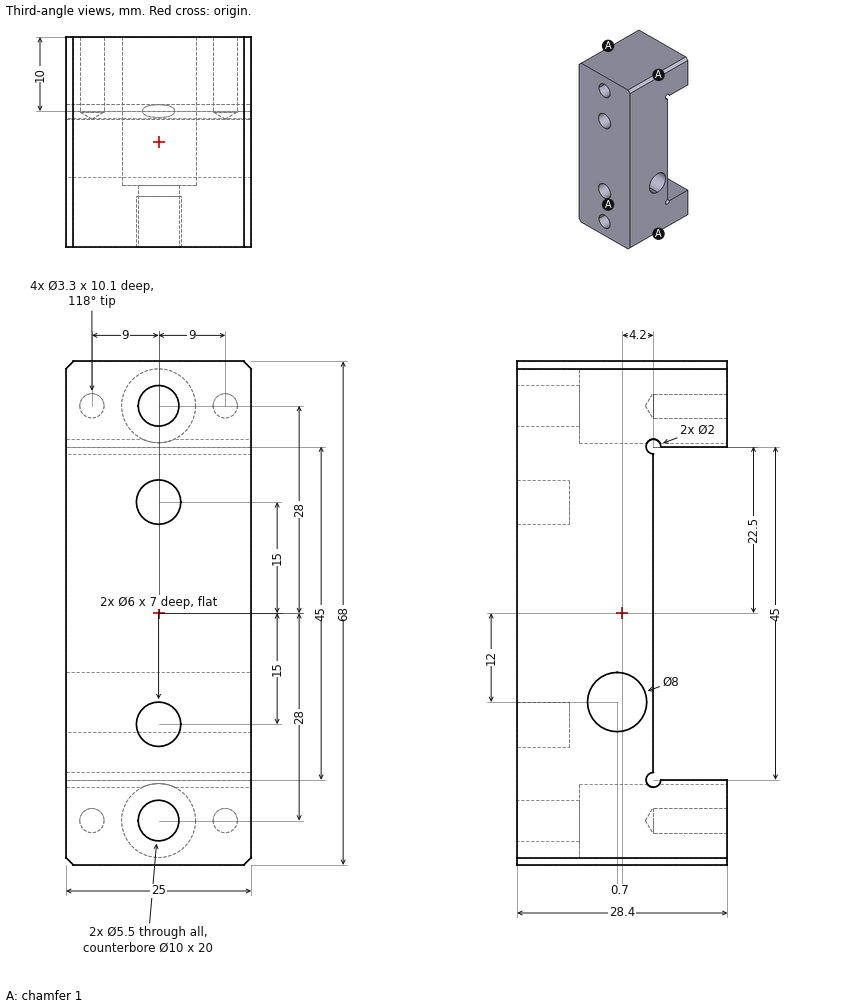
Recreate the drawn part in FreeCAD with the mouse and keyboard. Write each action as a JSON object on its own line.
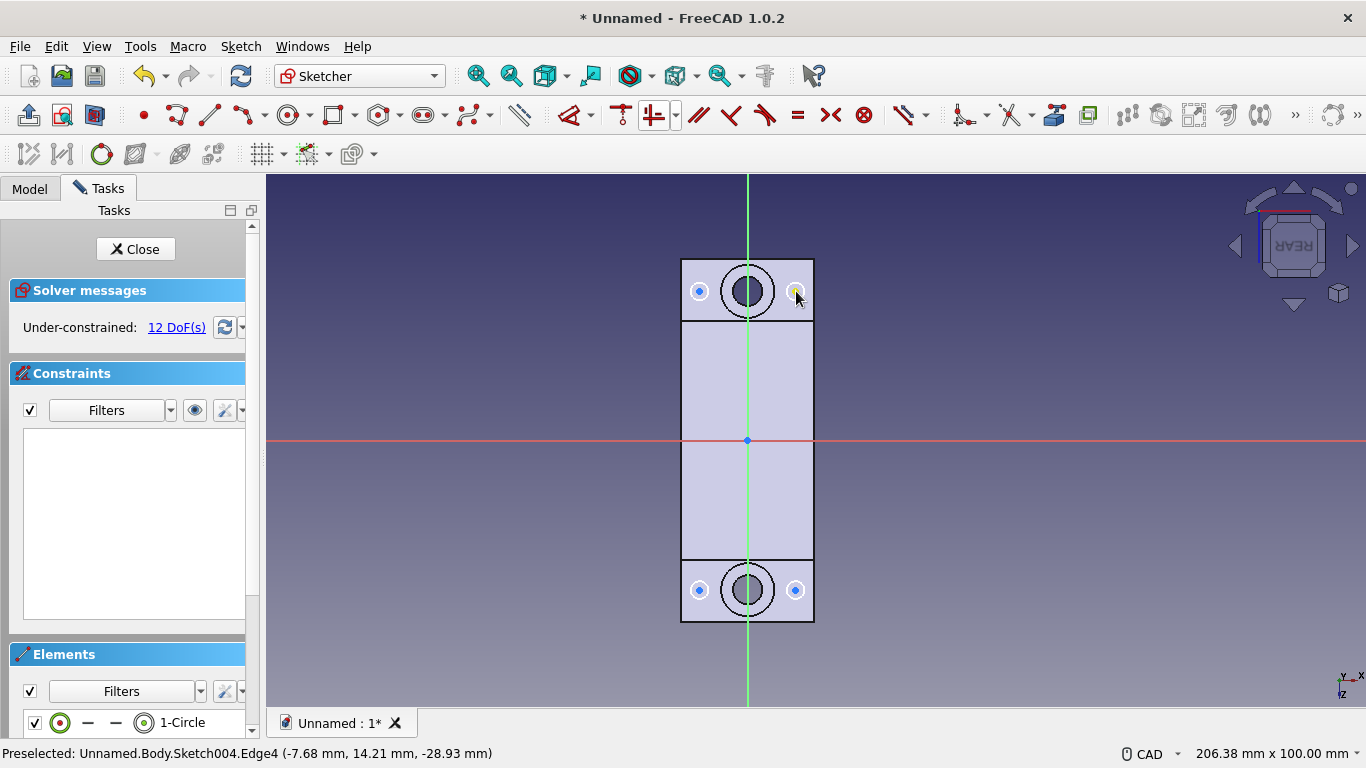
{"action": "scroll", "coordinate": [706, 584], "scroll_direction": "up", "scroll_amount": 3}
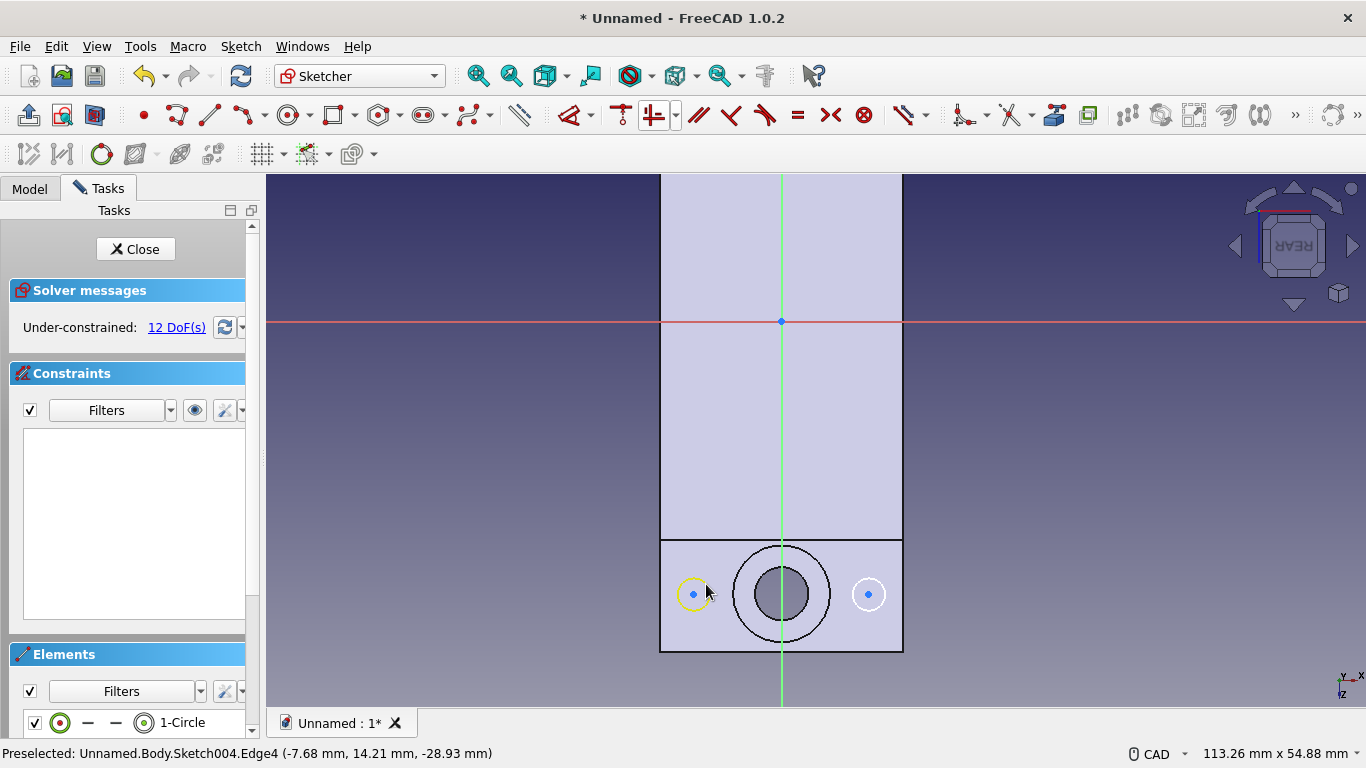
{"action": "left_click", "coordinate": [705, 583]}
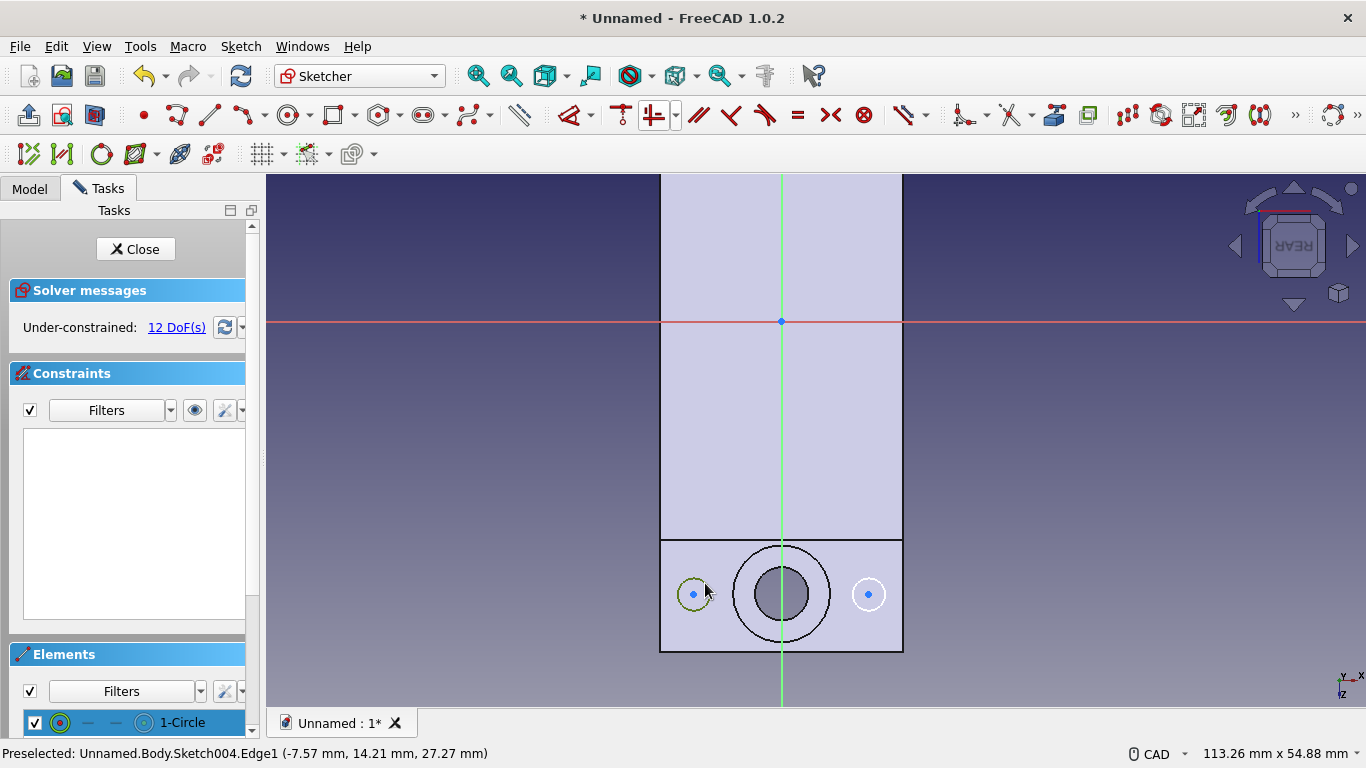
{"action": "left_click", "coordinate": [880, 583]}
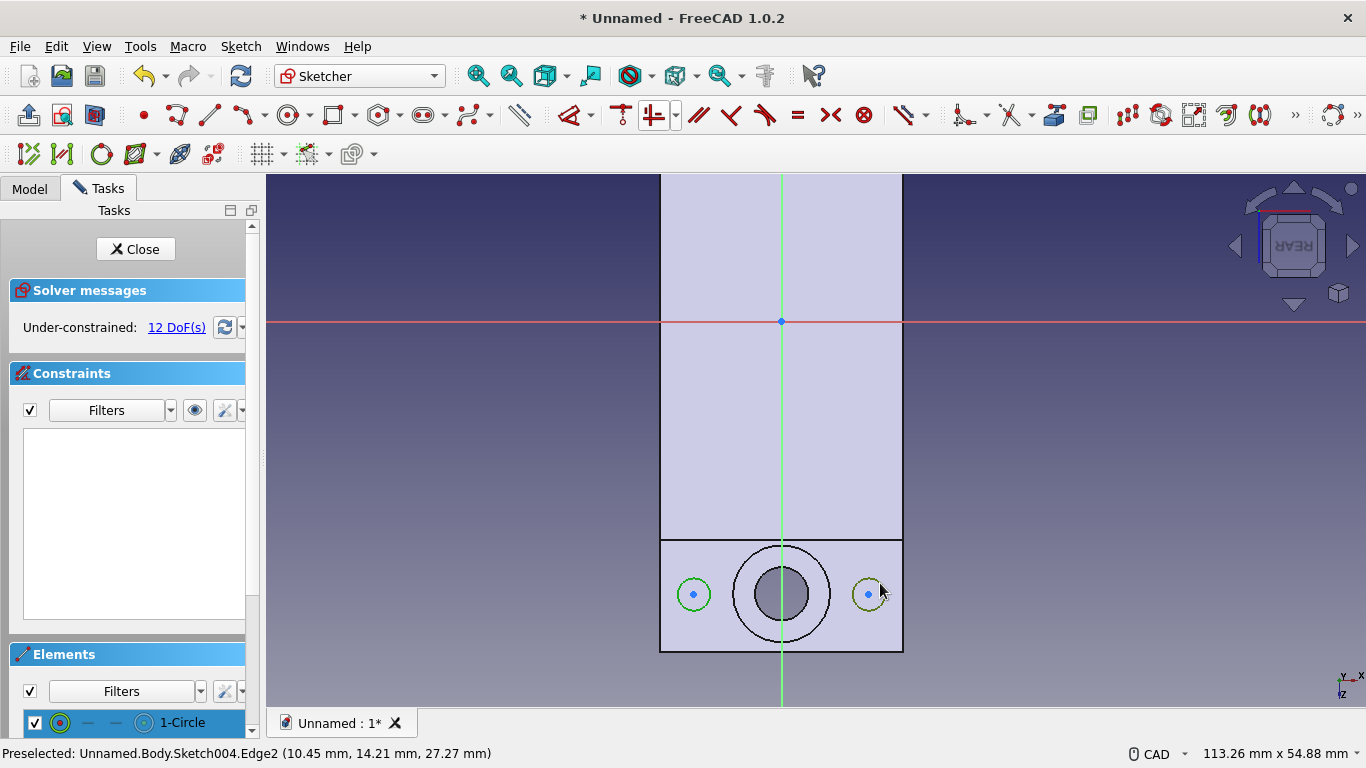
{"action": "scroll", "coordinate": [706, 585], "scroll_direction": "down", "scroll_amount": 3}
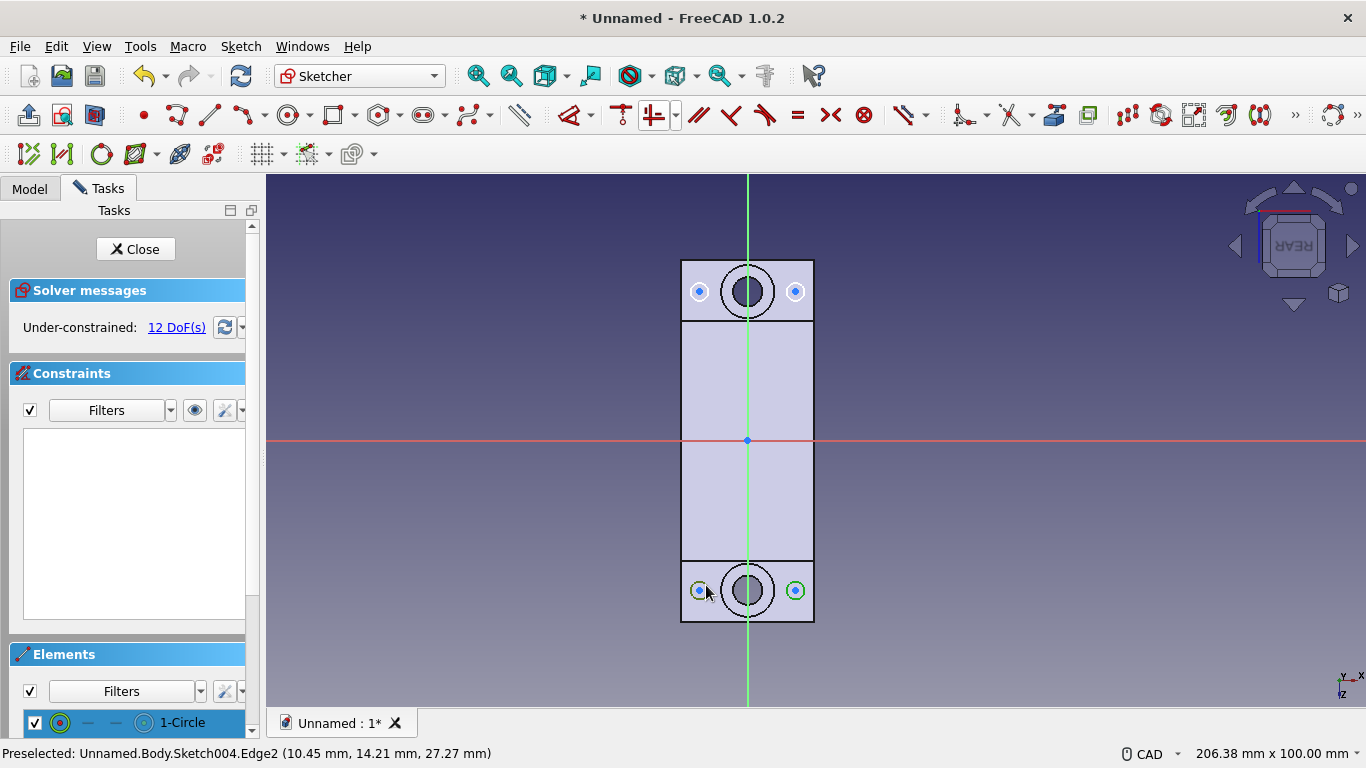
{"action": "scroll", "coordinate": [802, 286], "scroll_direction": "up", "scroll_amount": 3}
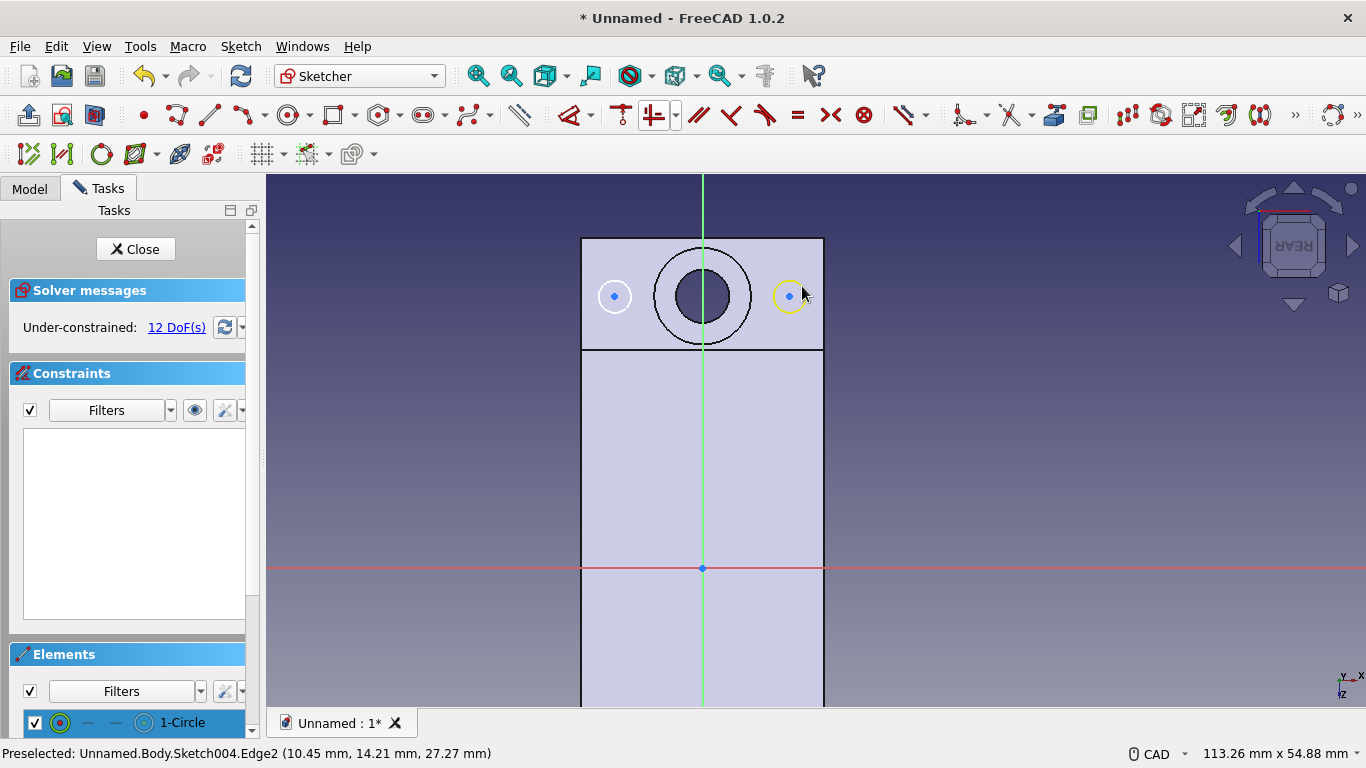
{"action": "left_click", "coordinate": [801, 285]}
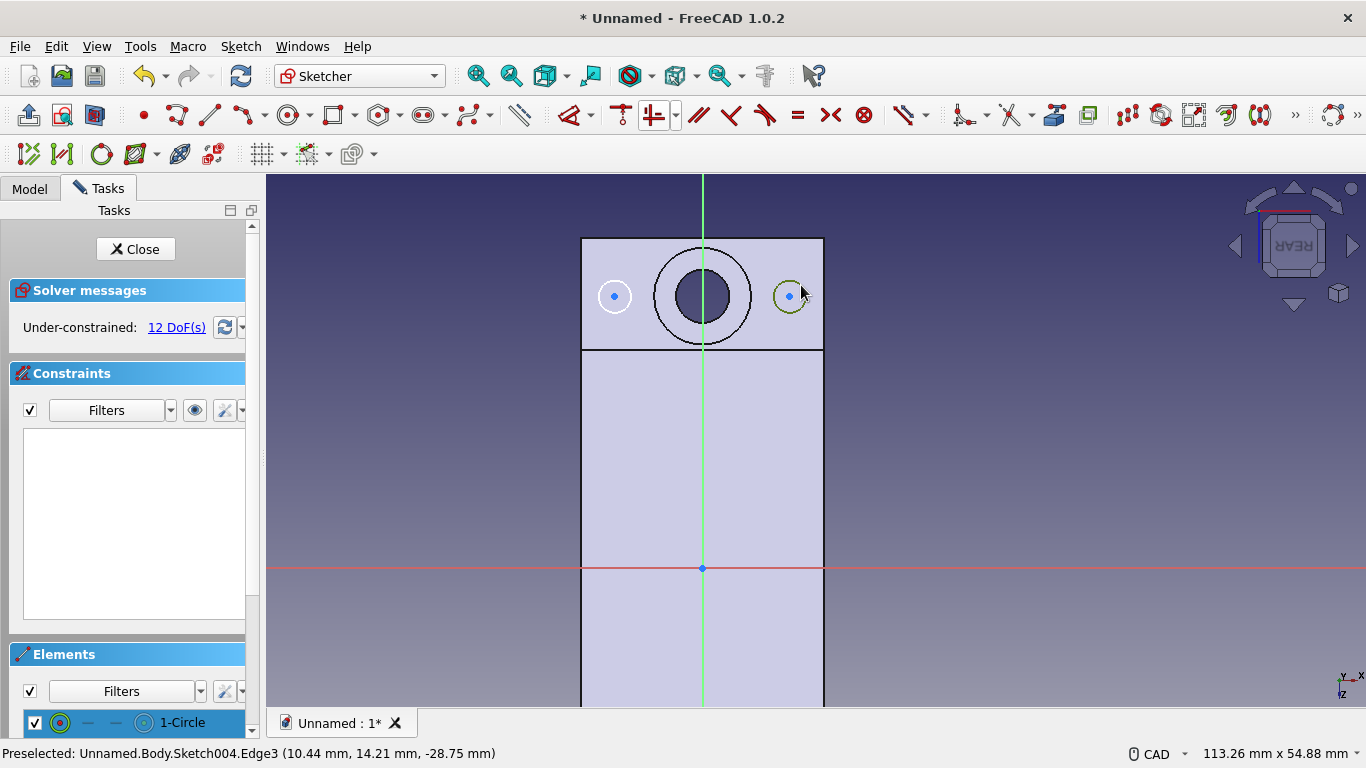
{"action": "left_click", "coordinate": [626, 285]}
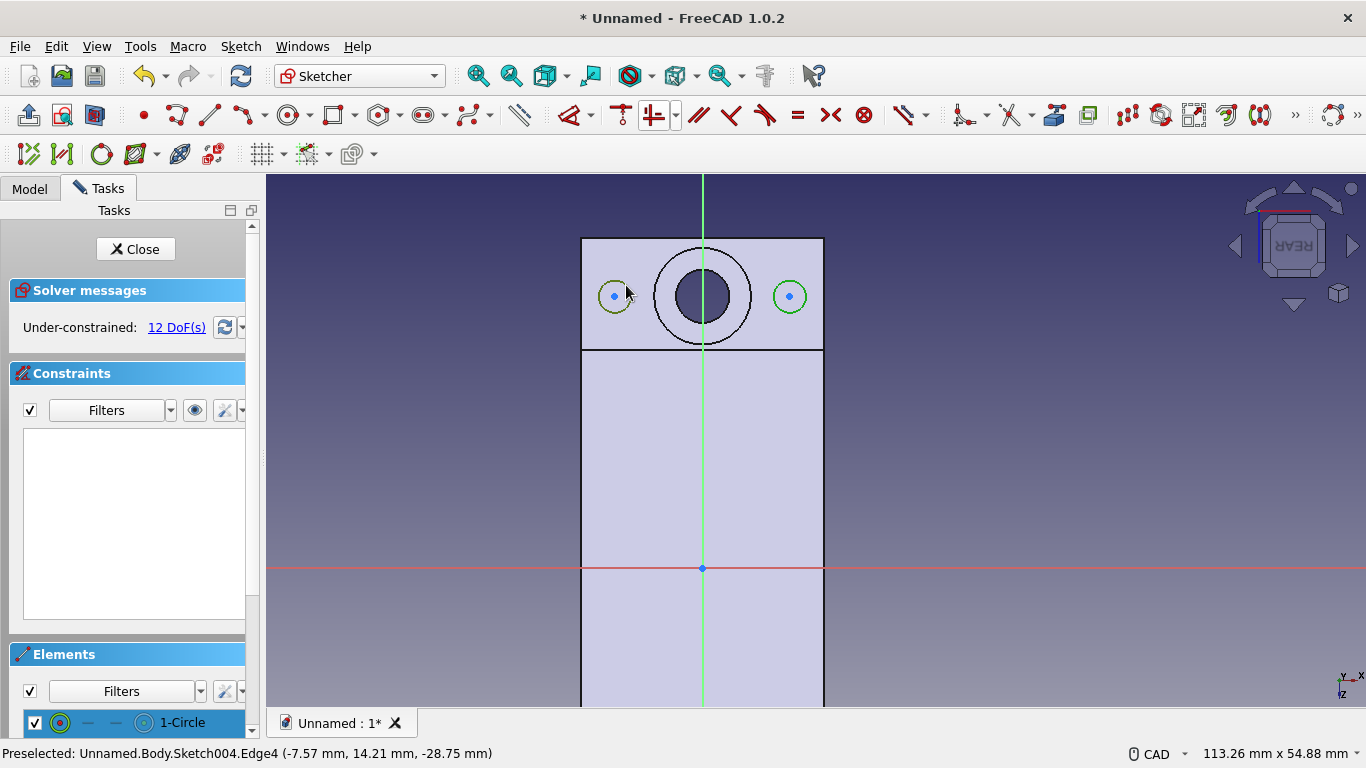
{"action": "key", "text": "e"}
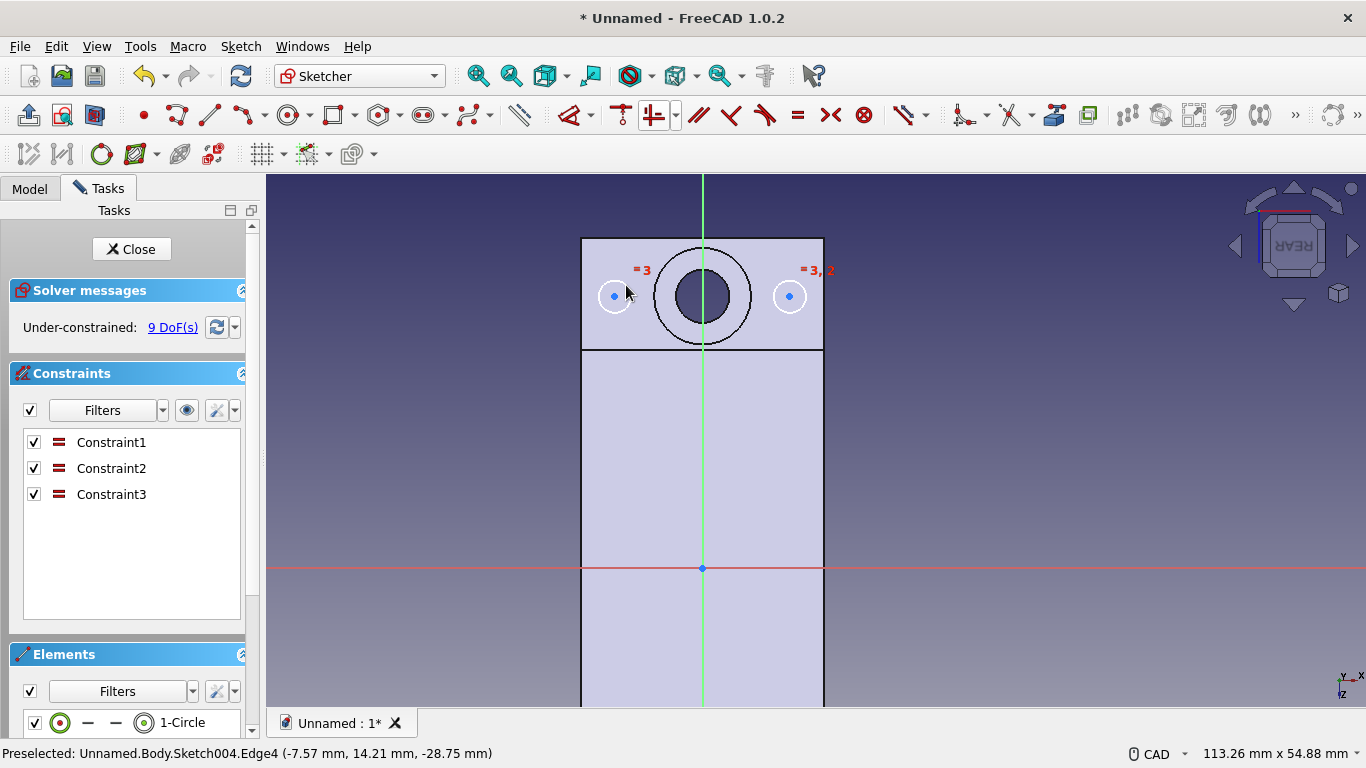
{"action": "scroll", "coordinate": [802, 285], "scroll_direction": "down", "scroll_amount": 3}